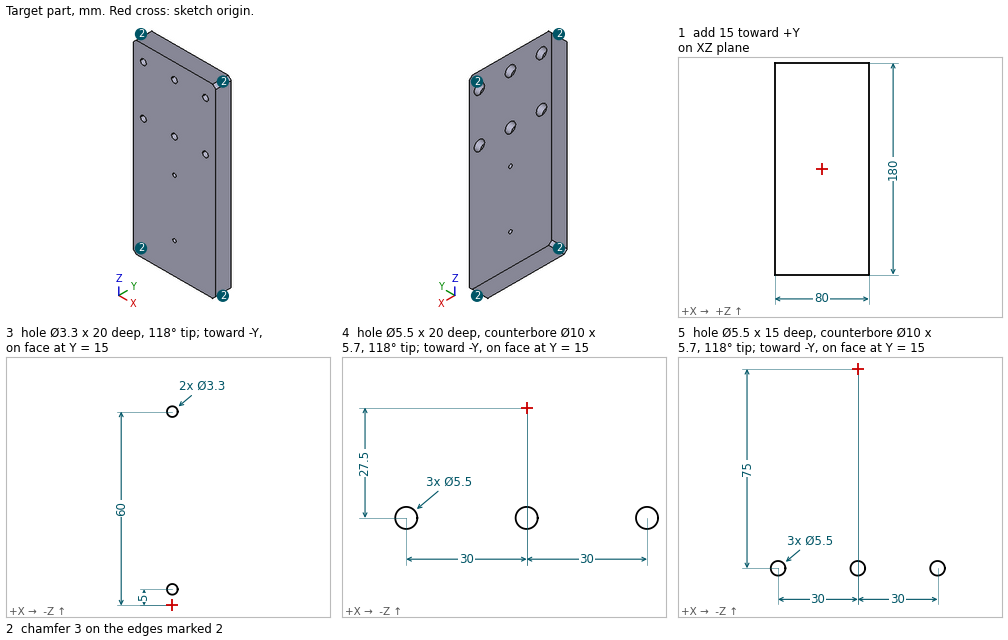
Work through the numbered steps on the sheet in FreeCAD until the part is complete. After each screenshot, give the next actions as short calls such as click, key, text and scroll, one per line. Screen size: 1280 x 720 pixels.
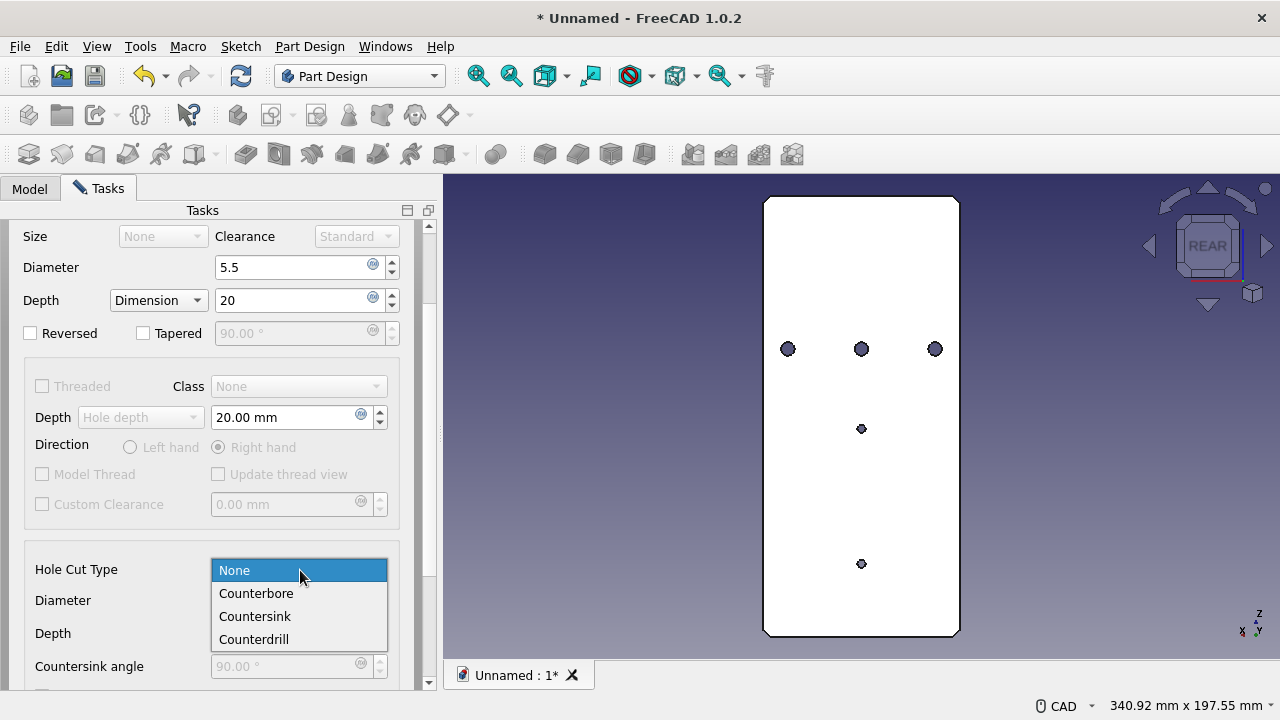
click(298, 594)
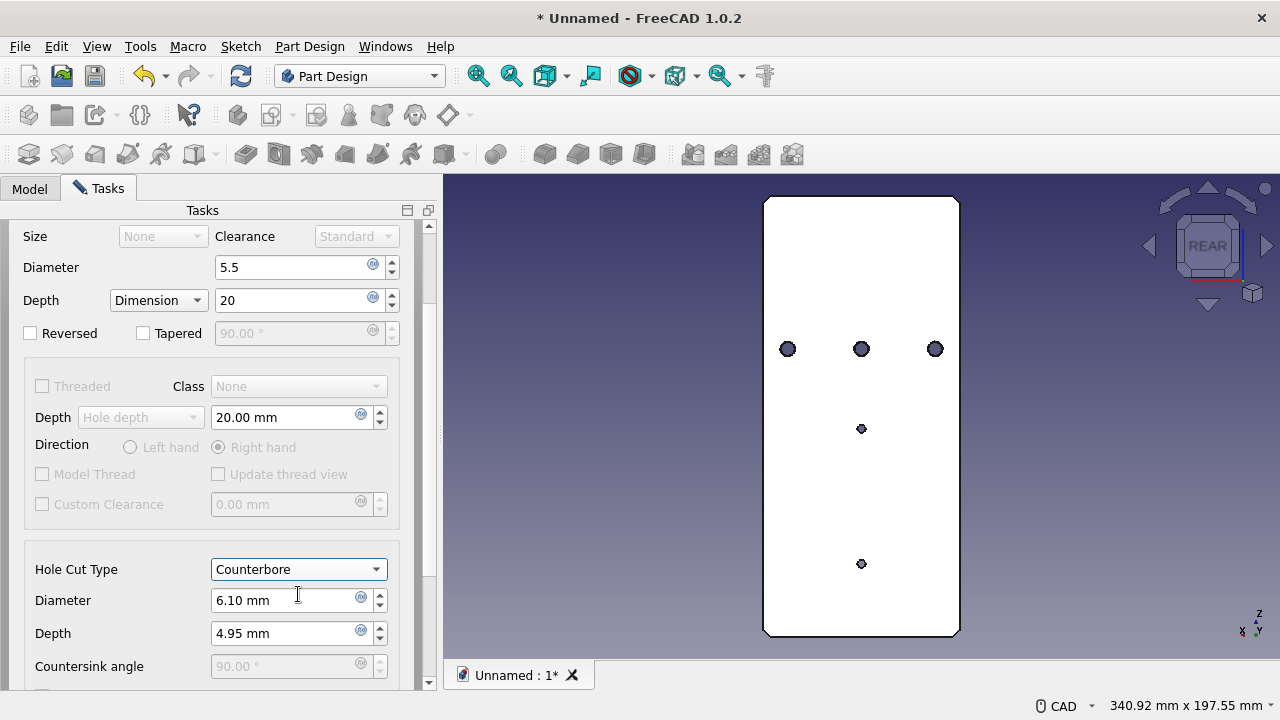
triple_click(292, 600)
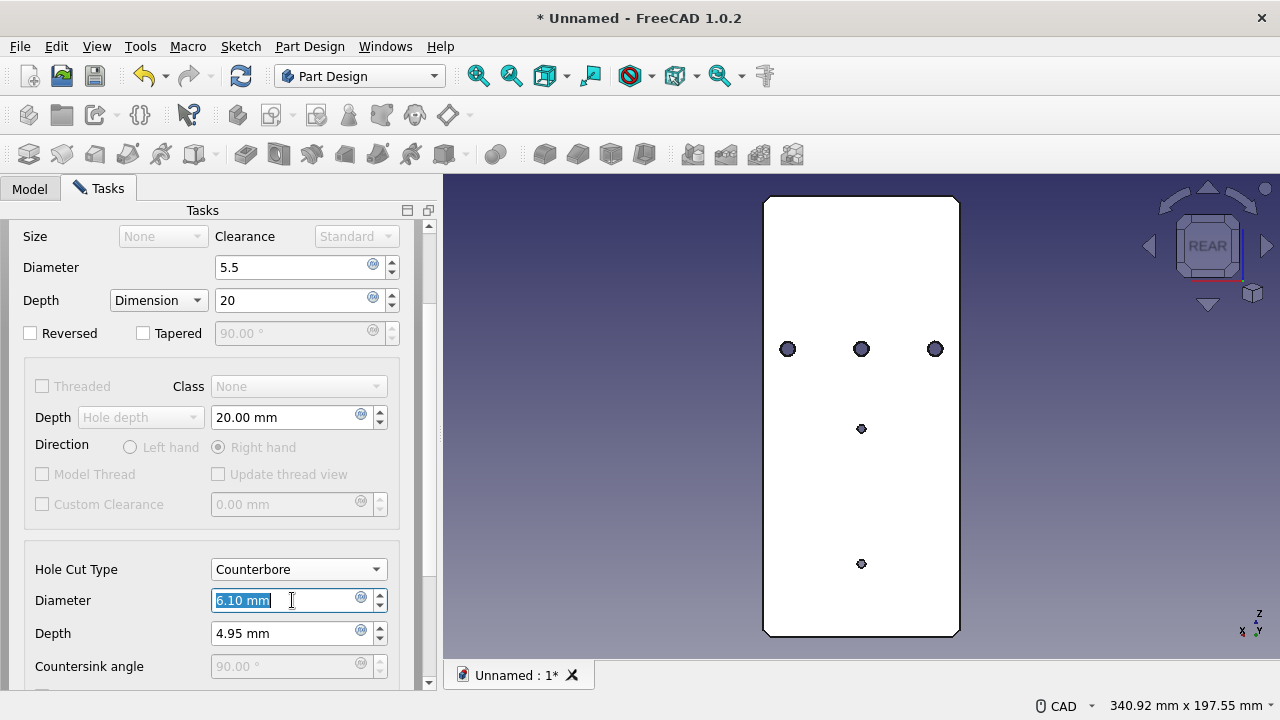
text(10)
key(Tab)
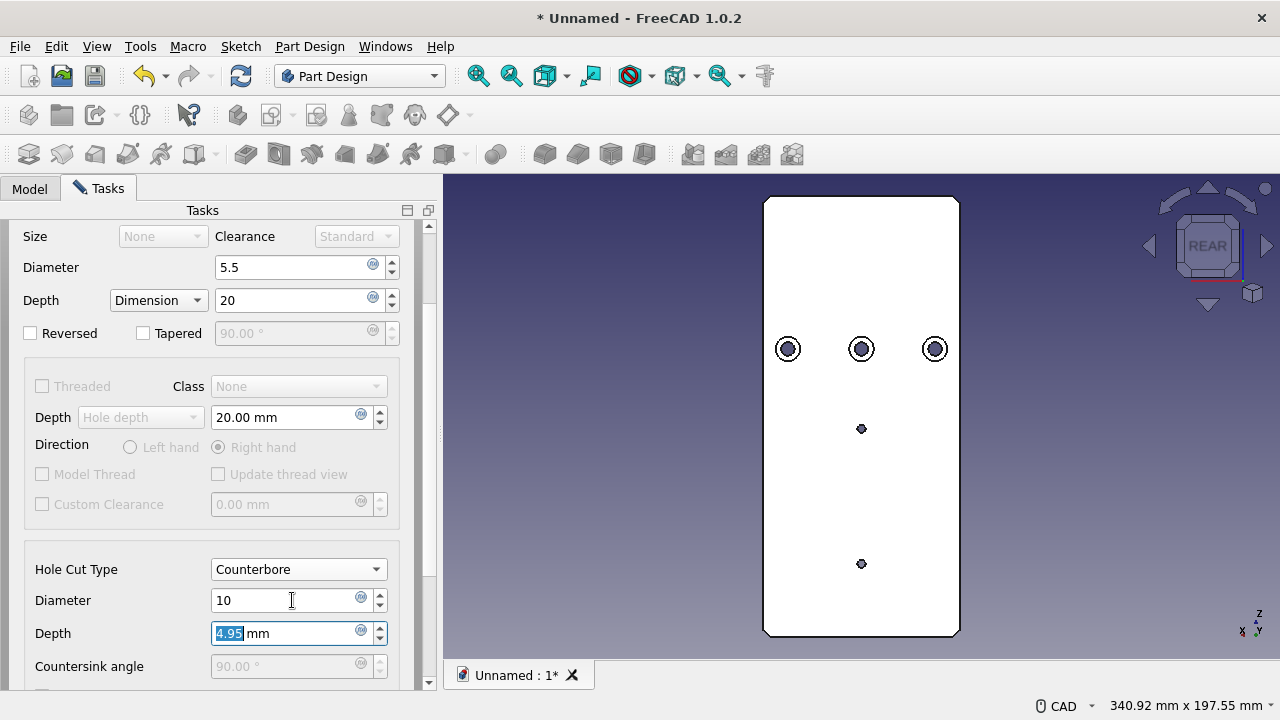
text(5.7)
key(Tab)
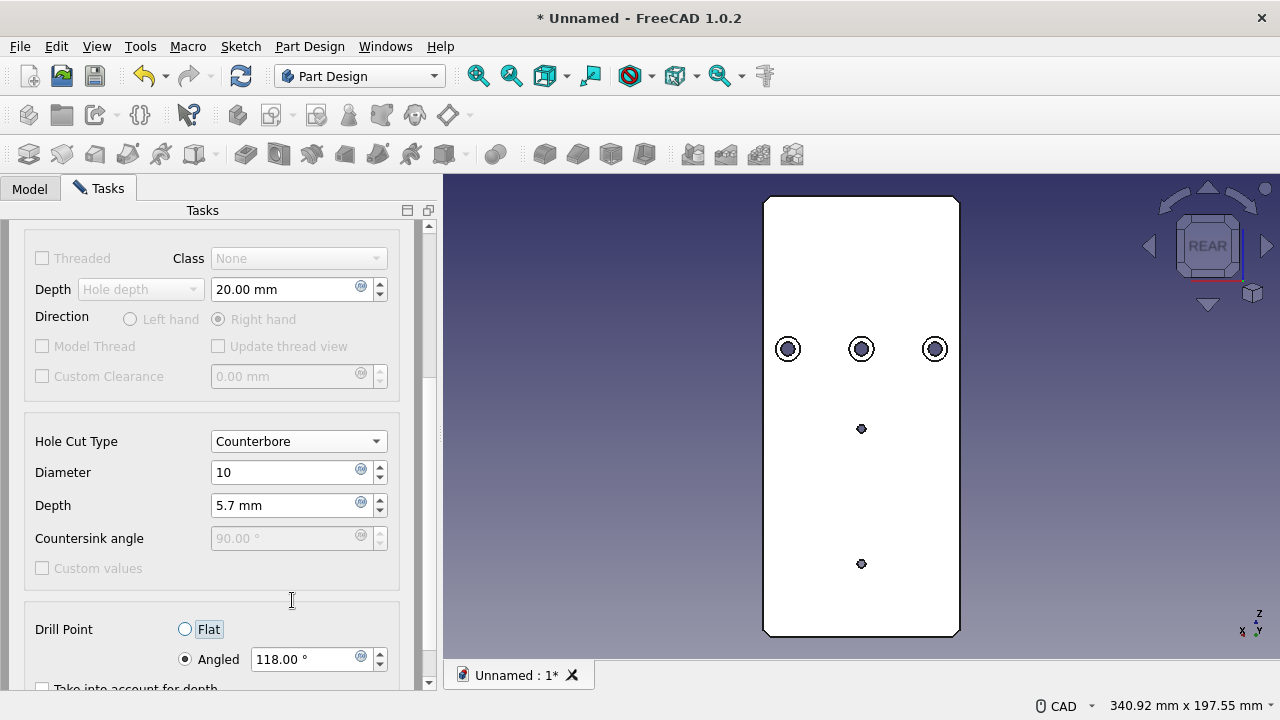
scroll(429, 455, up, 5)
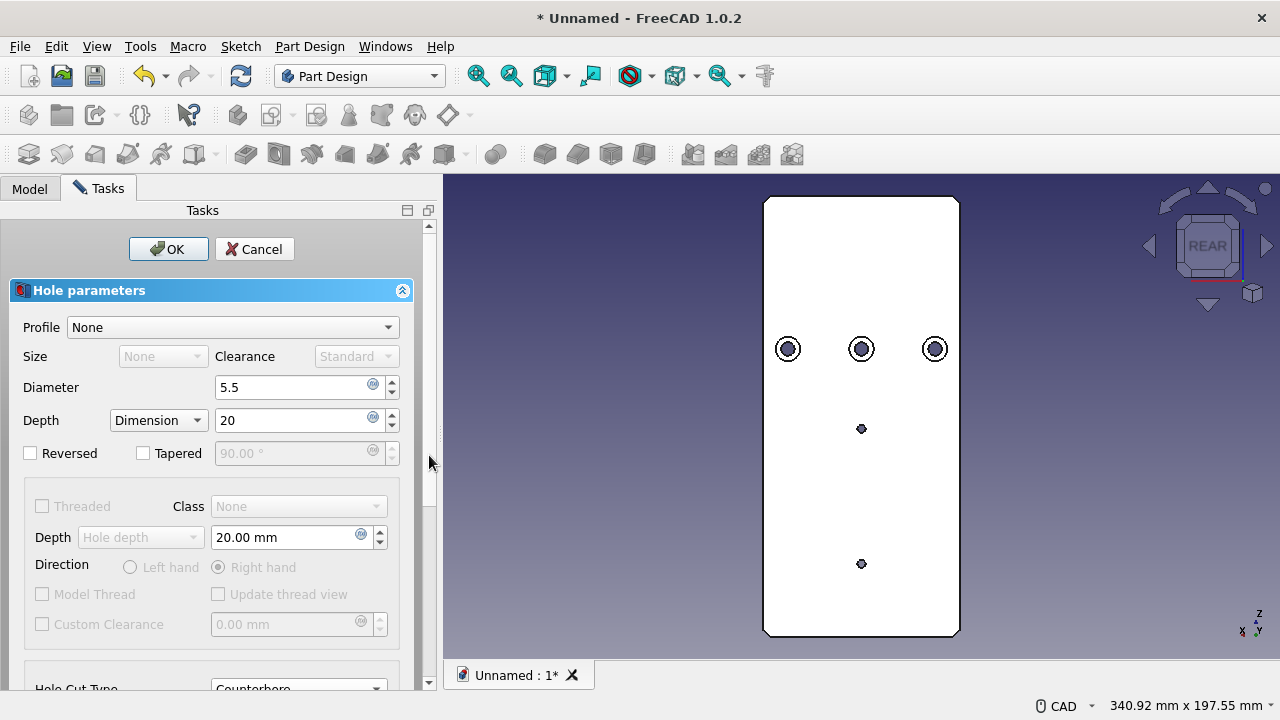
click(169, 249)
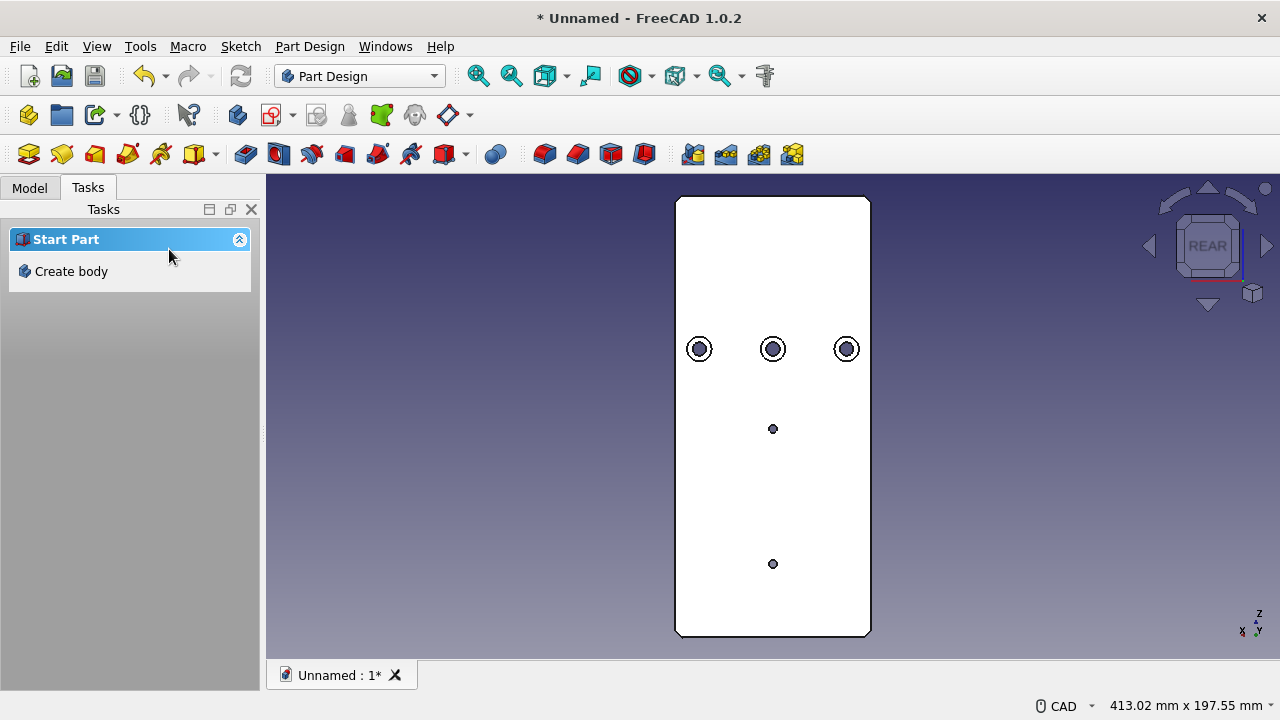
click(745, 479)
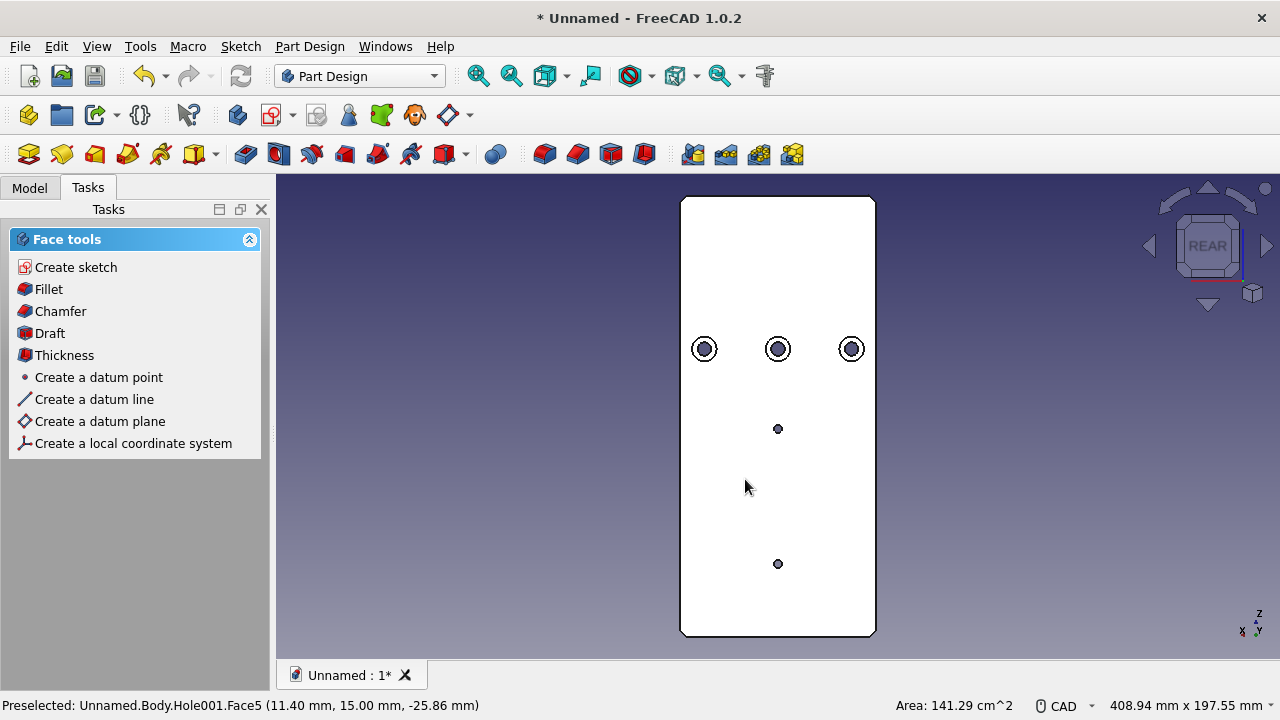
click(270, 116)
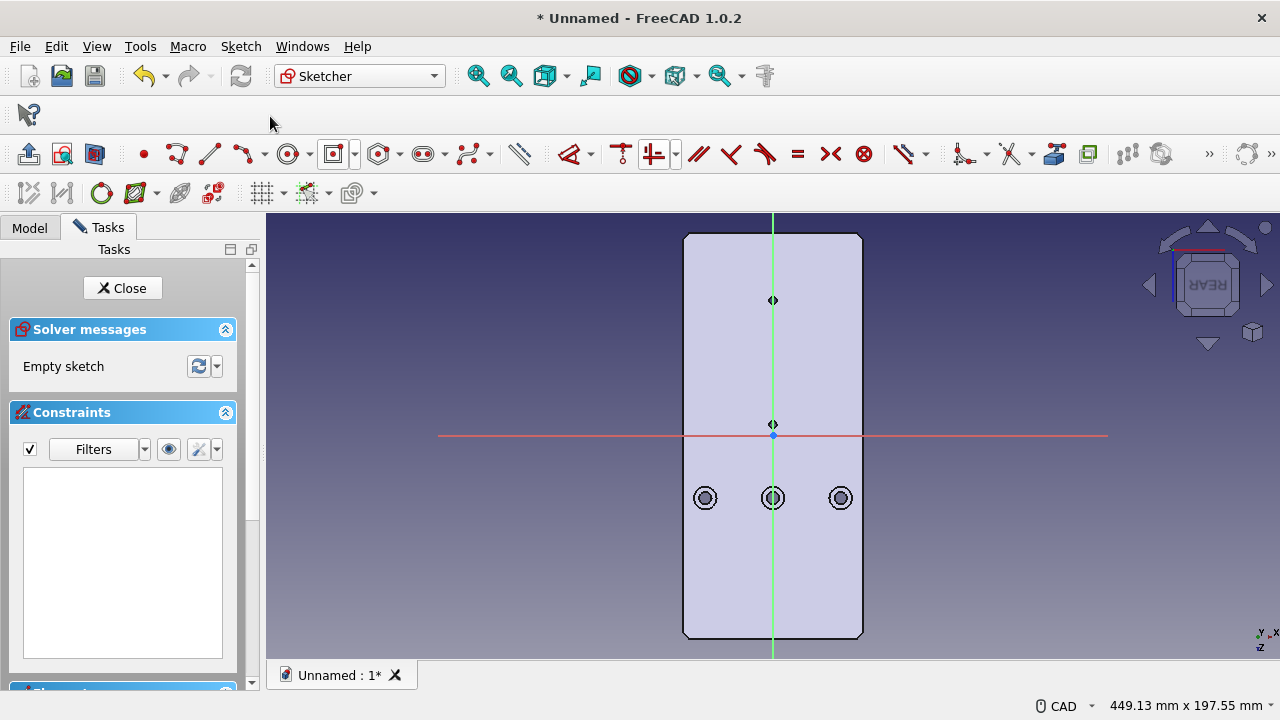
scroll(912, 631, up, 2)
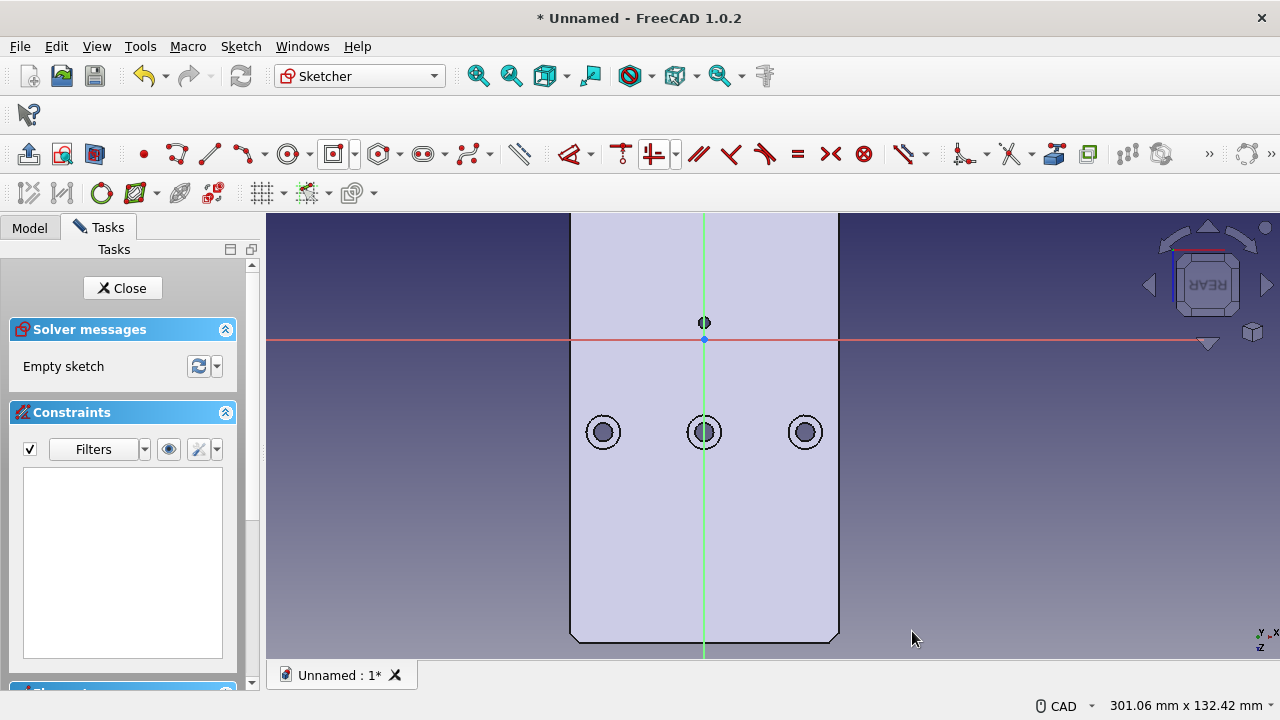
click(288, 154)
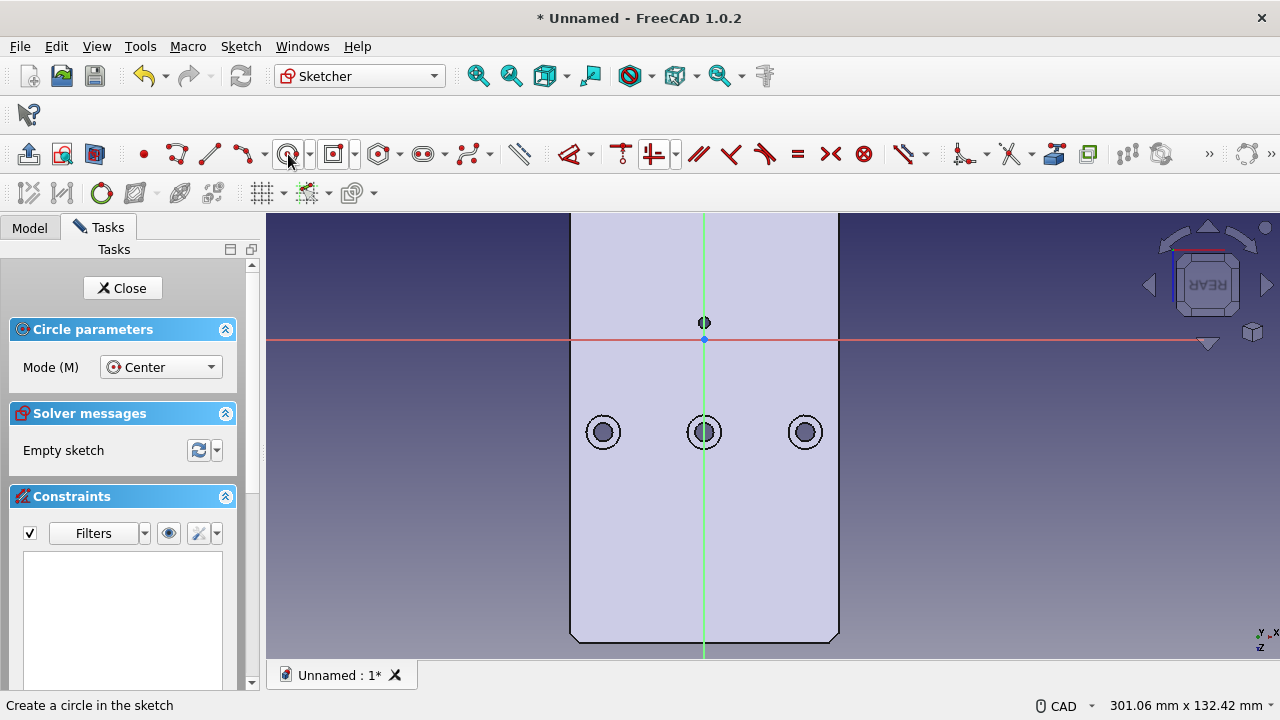
scroll(603, 592, up, 5)